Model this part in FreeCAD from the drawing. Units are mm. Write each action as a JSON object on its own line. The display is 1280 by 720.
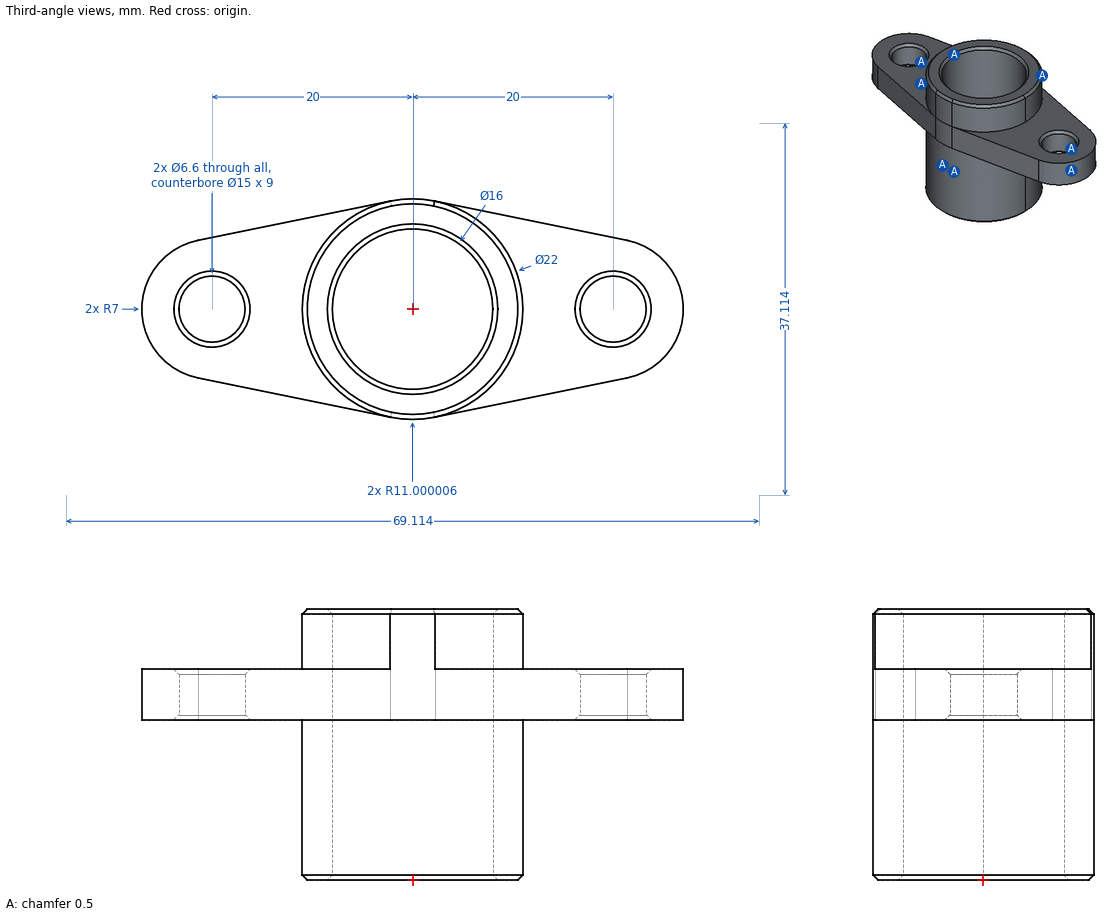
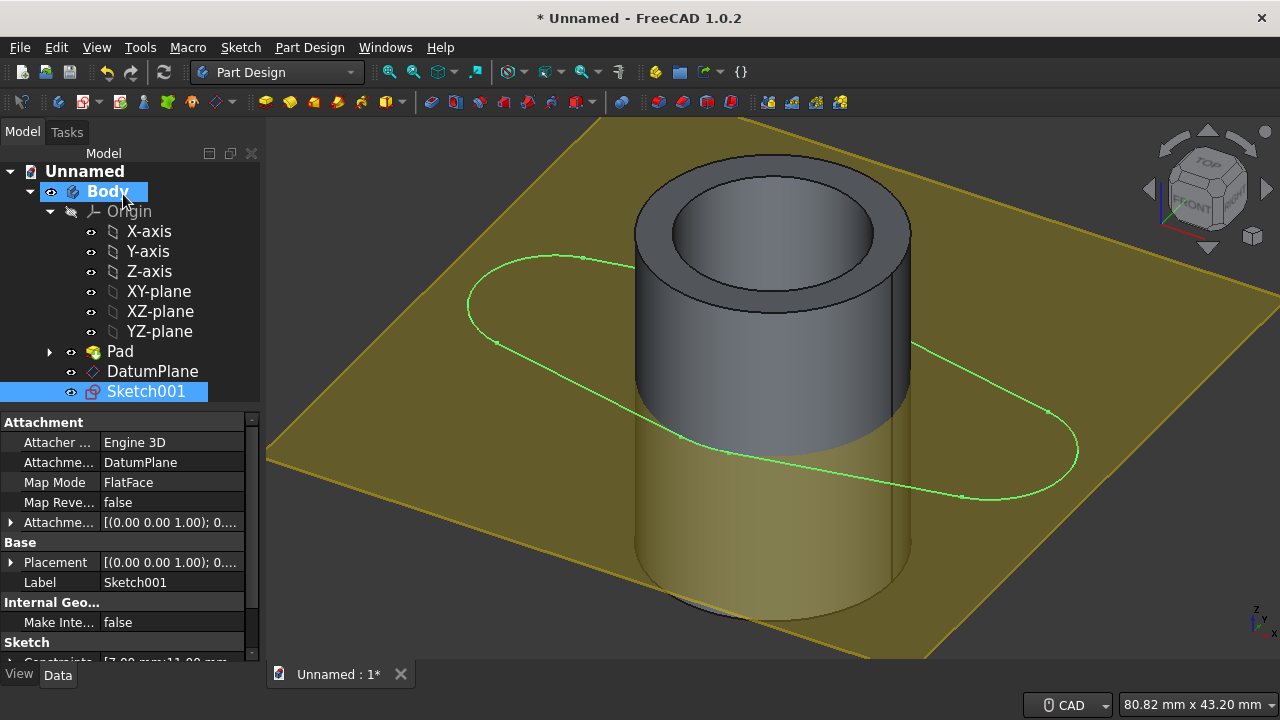
{"action": "left_click", "coordinate": [266, 102]}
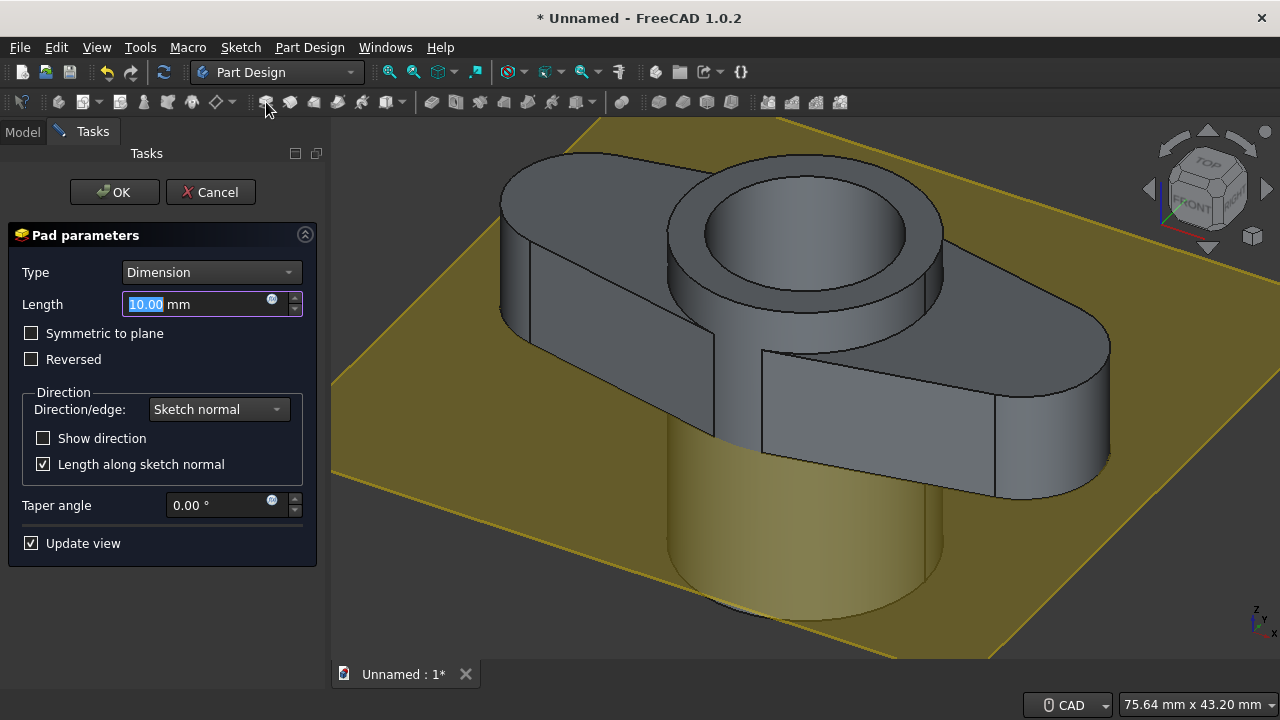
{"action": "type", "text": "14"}
{"action": "key", "text": "Tab"}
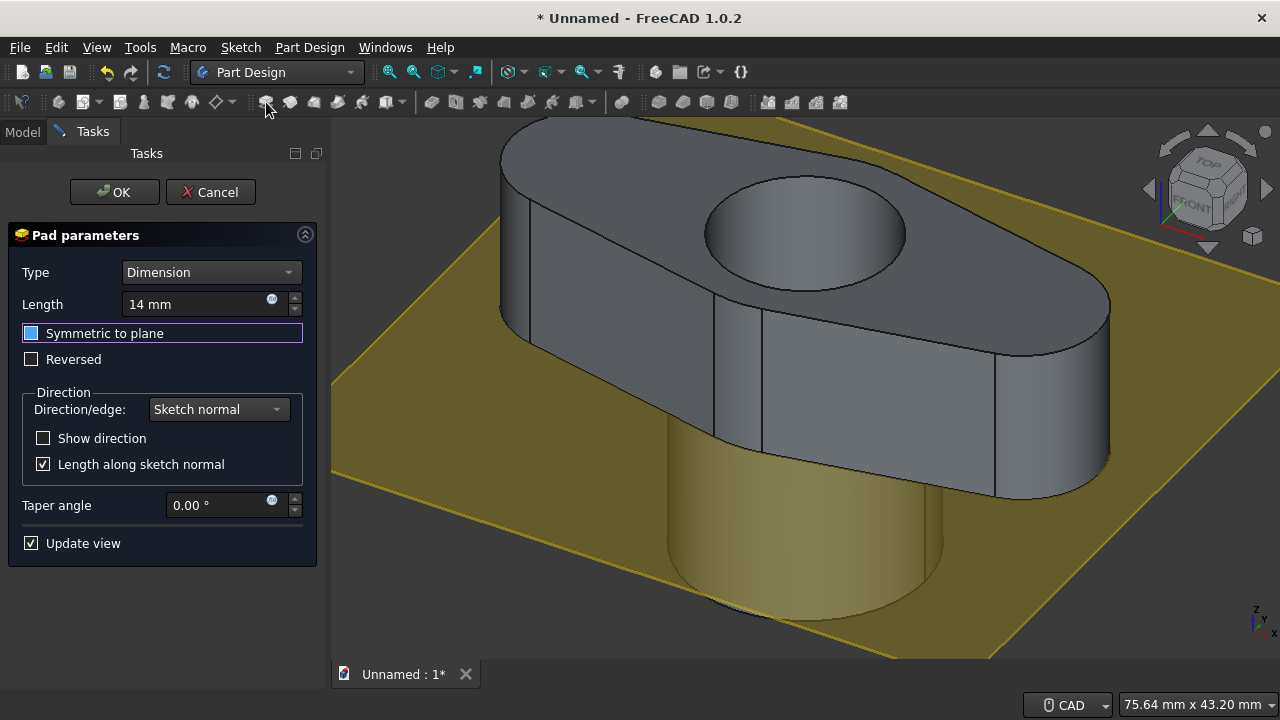
{"action": "left_click", "coordinate": [115, 192]}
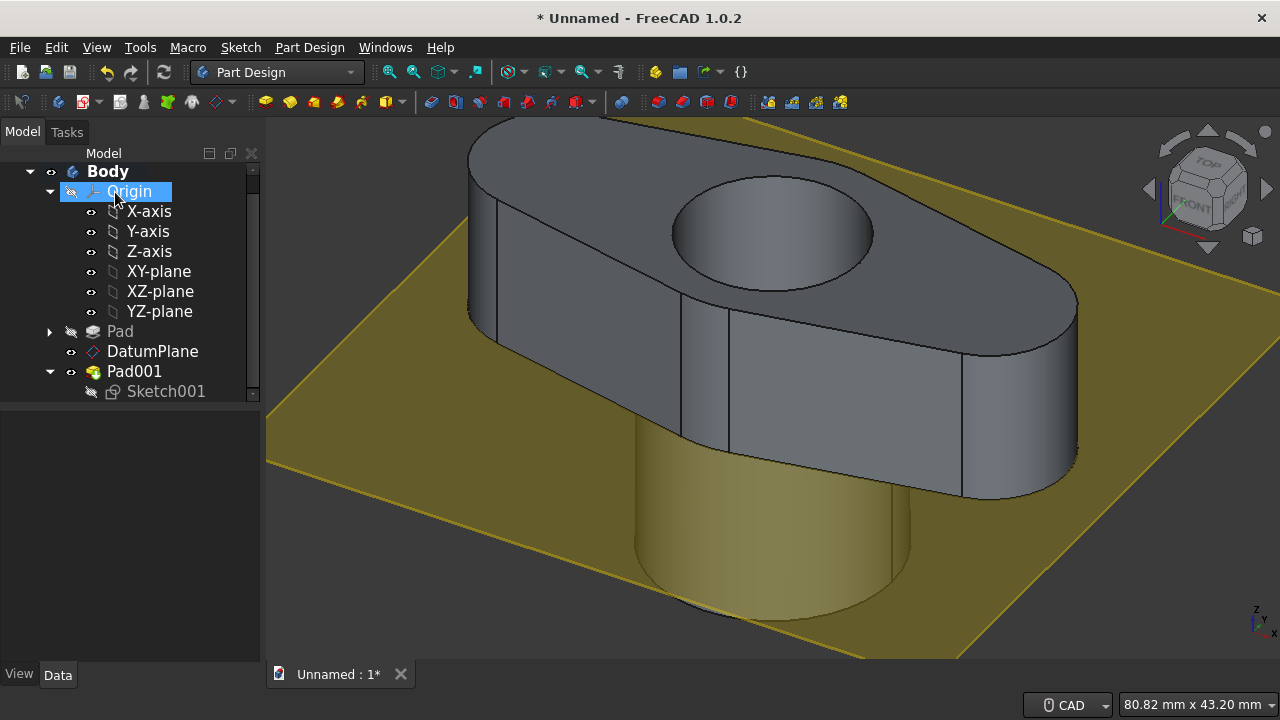
{"action": "left_click", "coordinate": [116, 352]}
{"action": "key", "text": "space"}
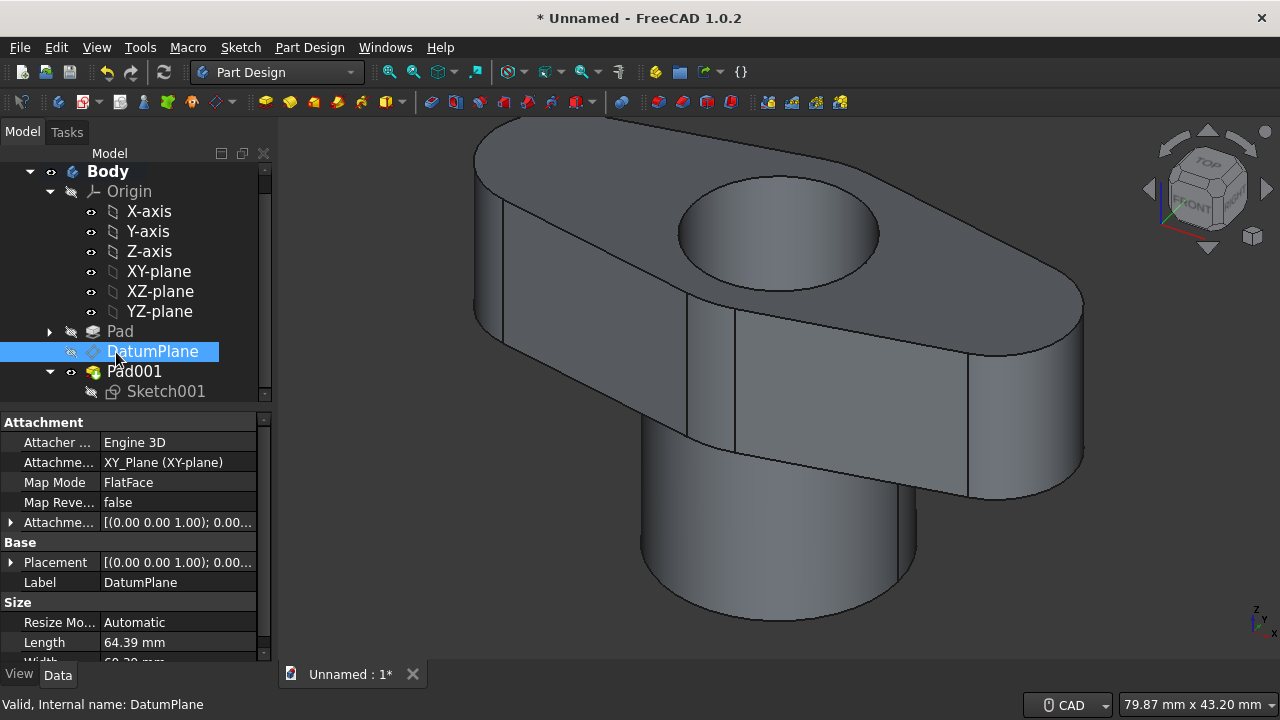
{"action": "left_click", "coordinate": [390, 72]}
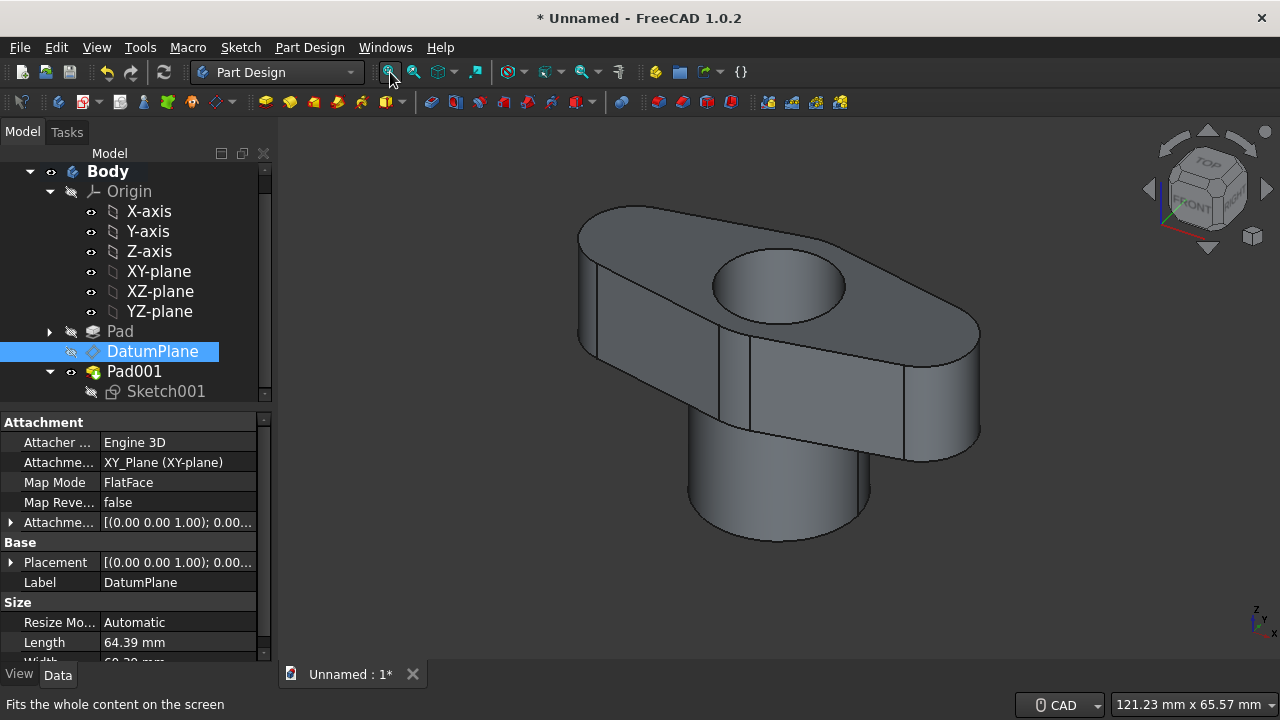
{"action": "left_click", "coordinate": [669, 249]}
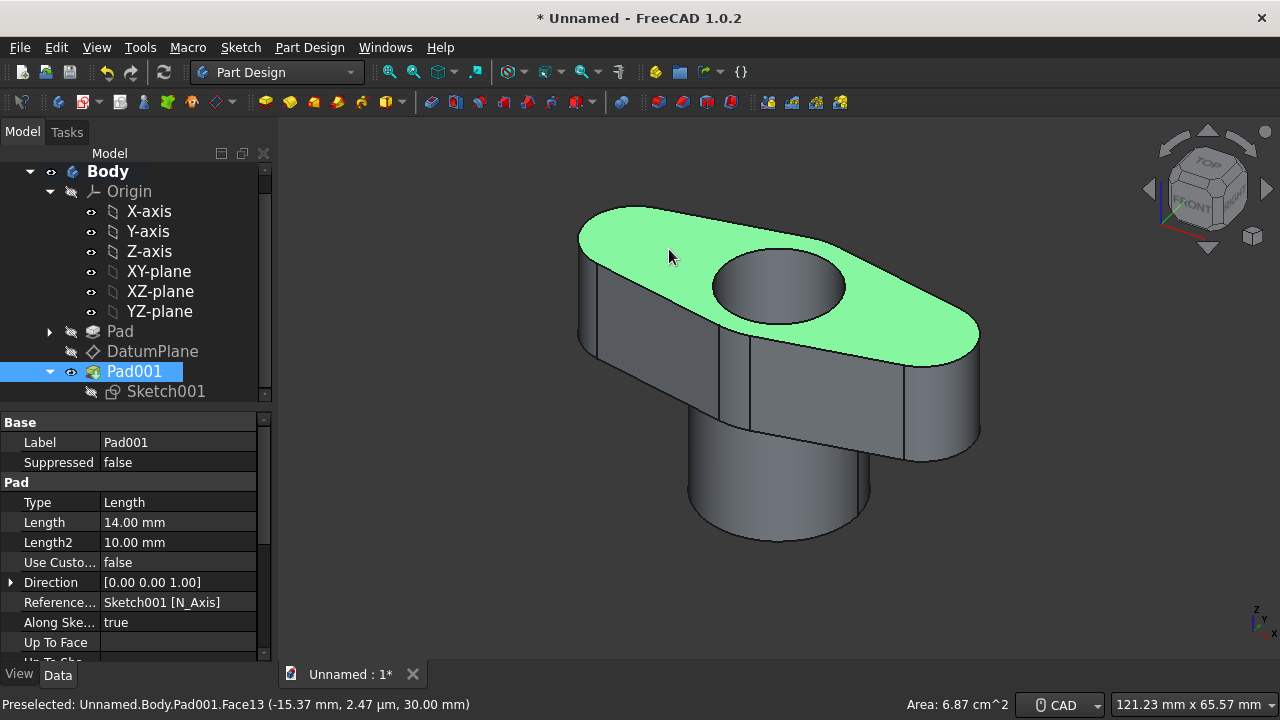
{"action": "left_click", "coordinate": [84, 102]}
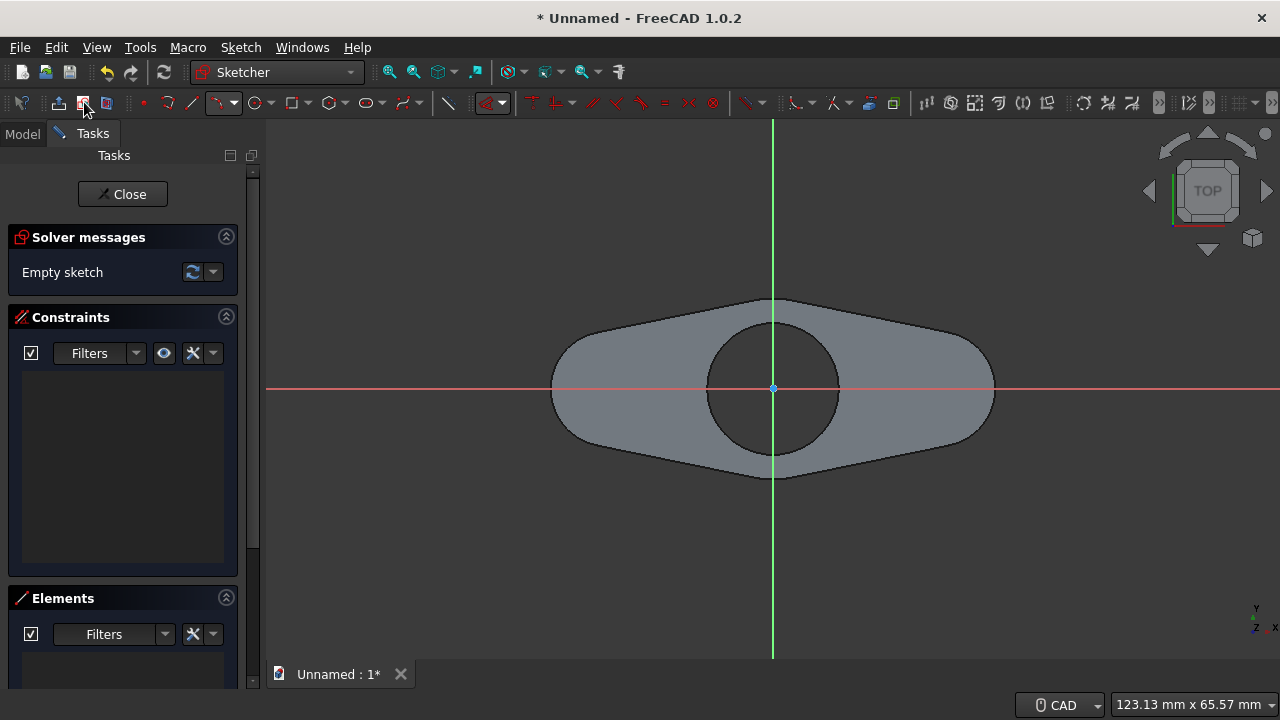
{"action": "scroll", "coordinate": [912, 389], "scroll_direction": "up", "scroll_amount": 2}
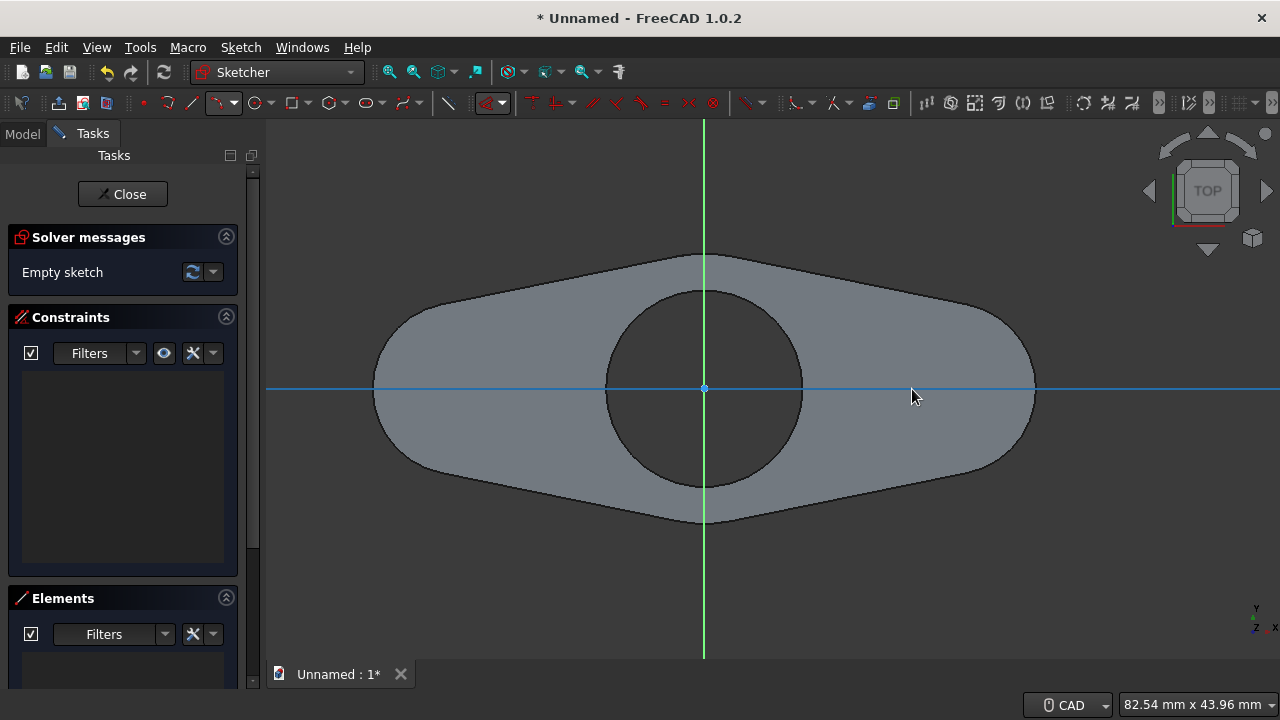
{"action": "left_click", "coordinate": [256, 104]}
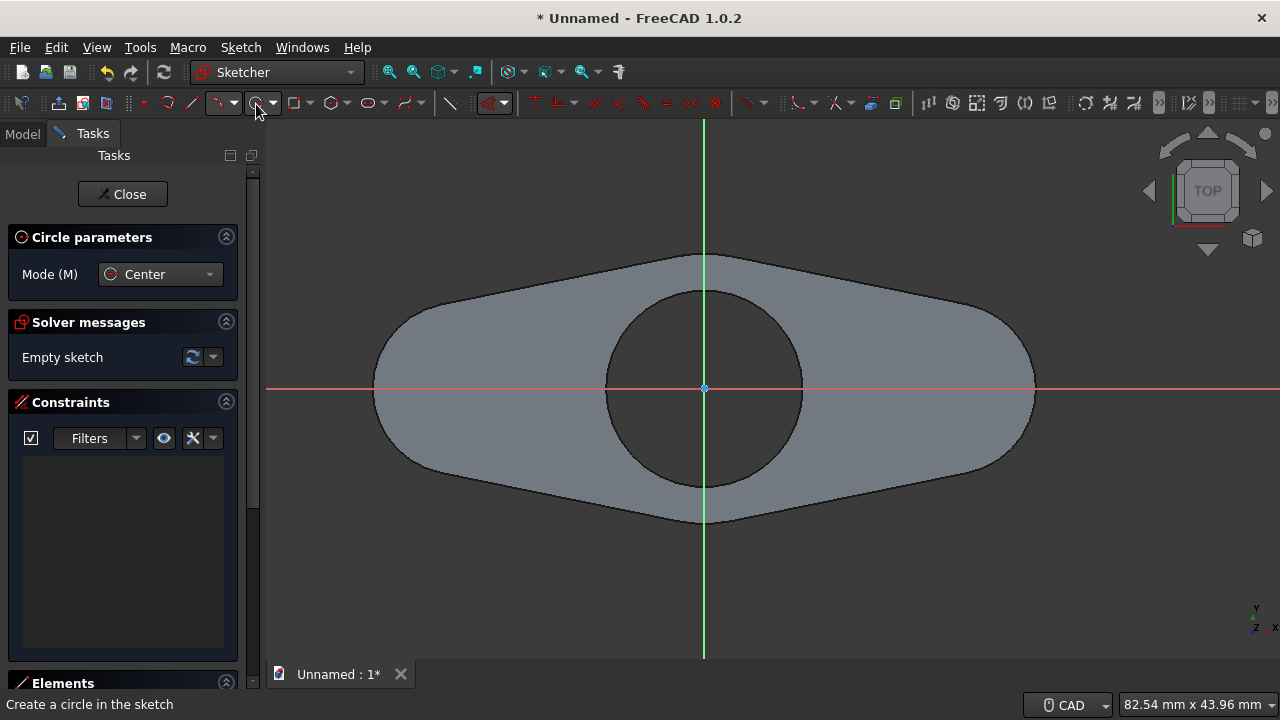
{"action": "left_click", "coordinate": [459, 389]}
{"action": "left_click", "coordinate": [487, 360]}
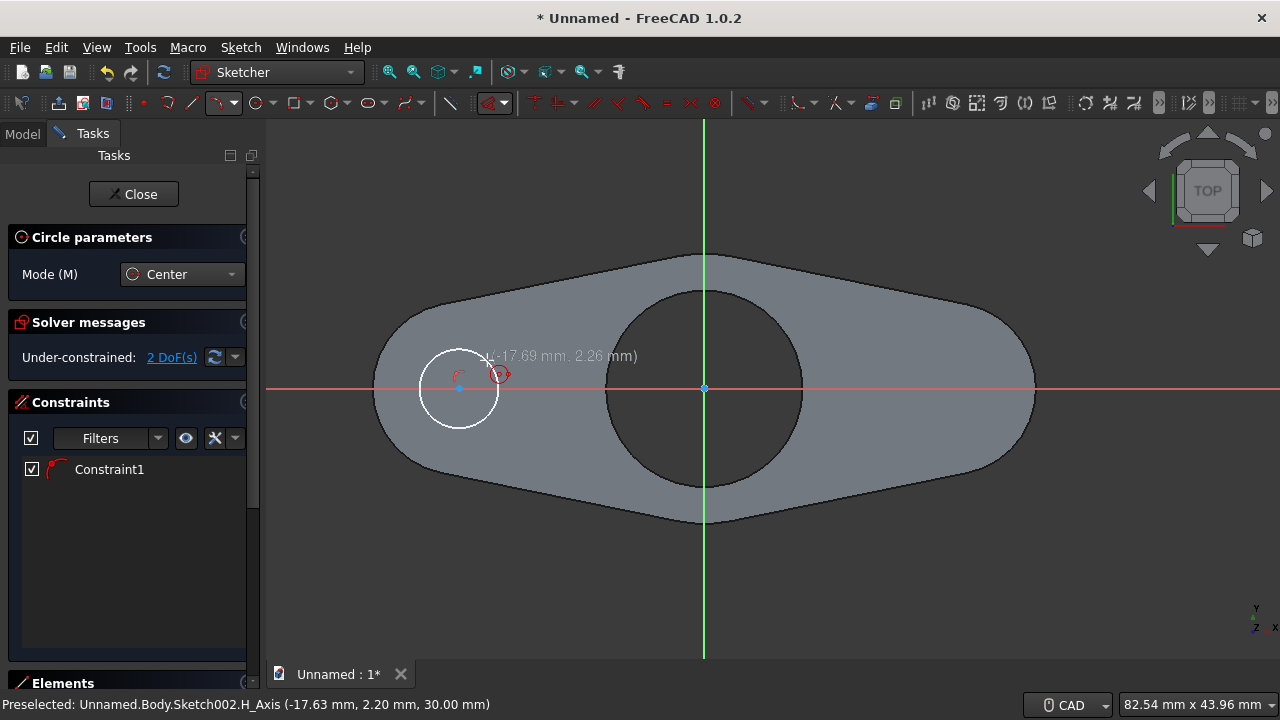
{"action": "left_click", "coordinate": [950, 389]}
{"action": "left_click", "coordinate": [979, 360]}
{"action": "key", "text": "Escape"}